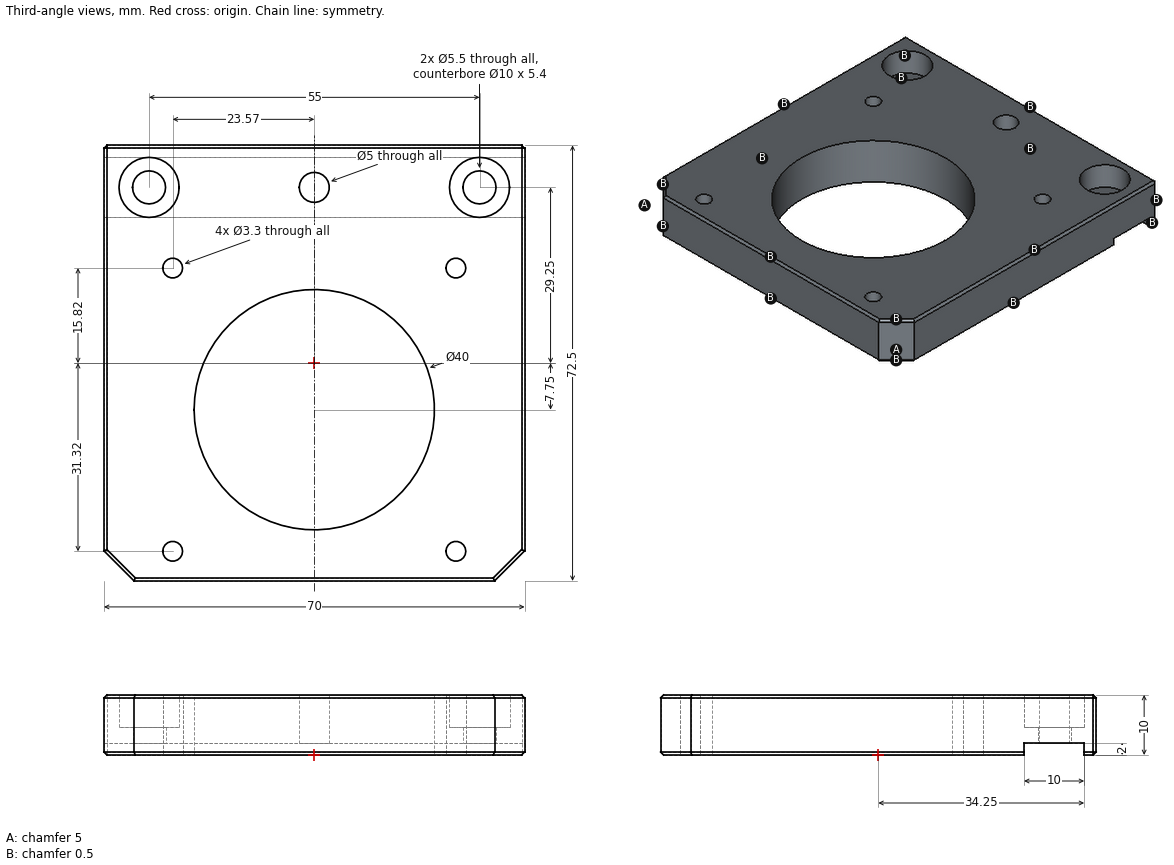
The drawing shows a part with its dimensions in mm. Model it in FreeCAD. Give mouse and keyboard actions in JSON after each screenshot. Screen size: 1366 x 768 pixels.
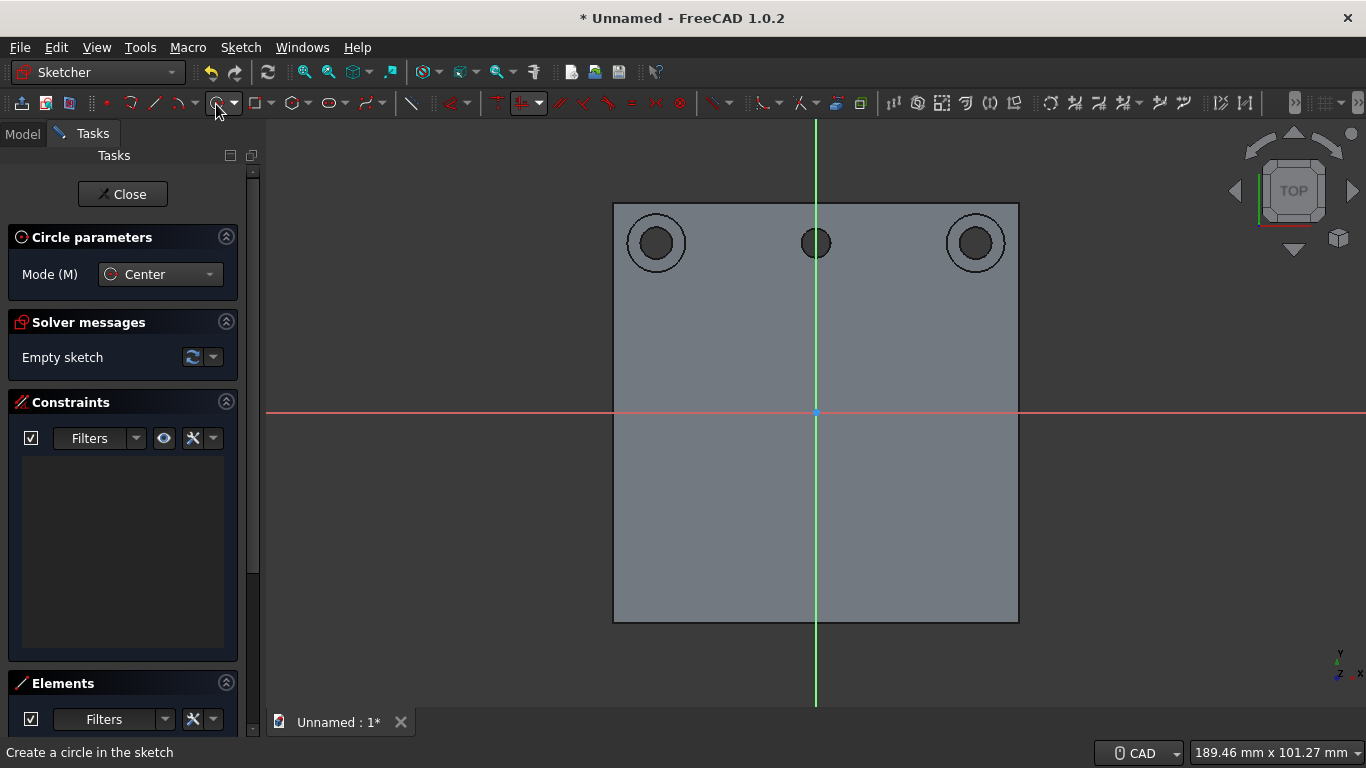
{"action": "scroll", "coordinate": [679, 321], "scroll_direction": "up", "scroll_amount": 5}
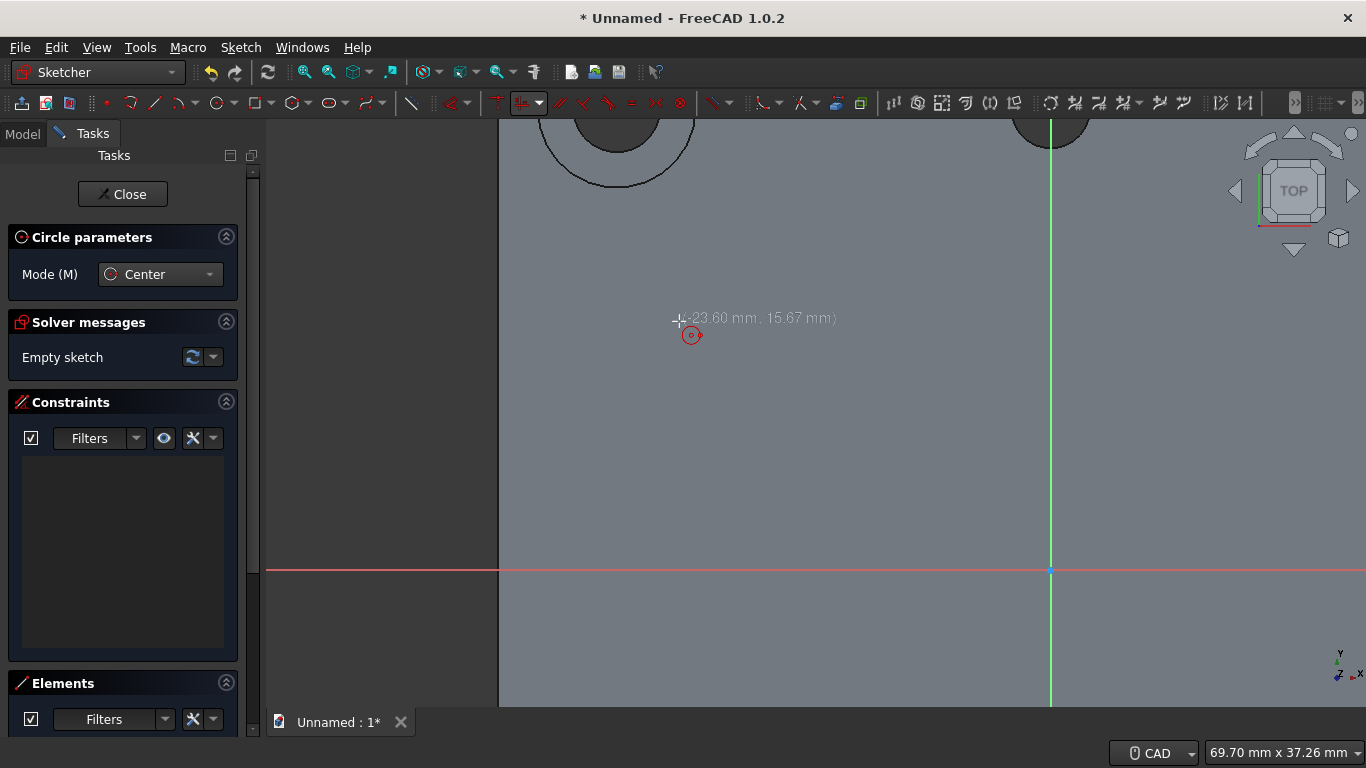
{"action": "left_click", "coordinate": [679, 321]}
{"action": "mouse_move", "coordinate": [697, 302]}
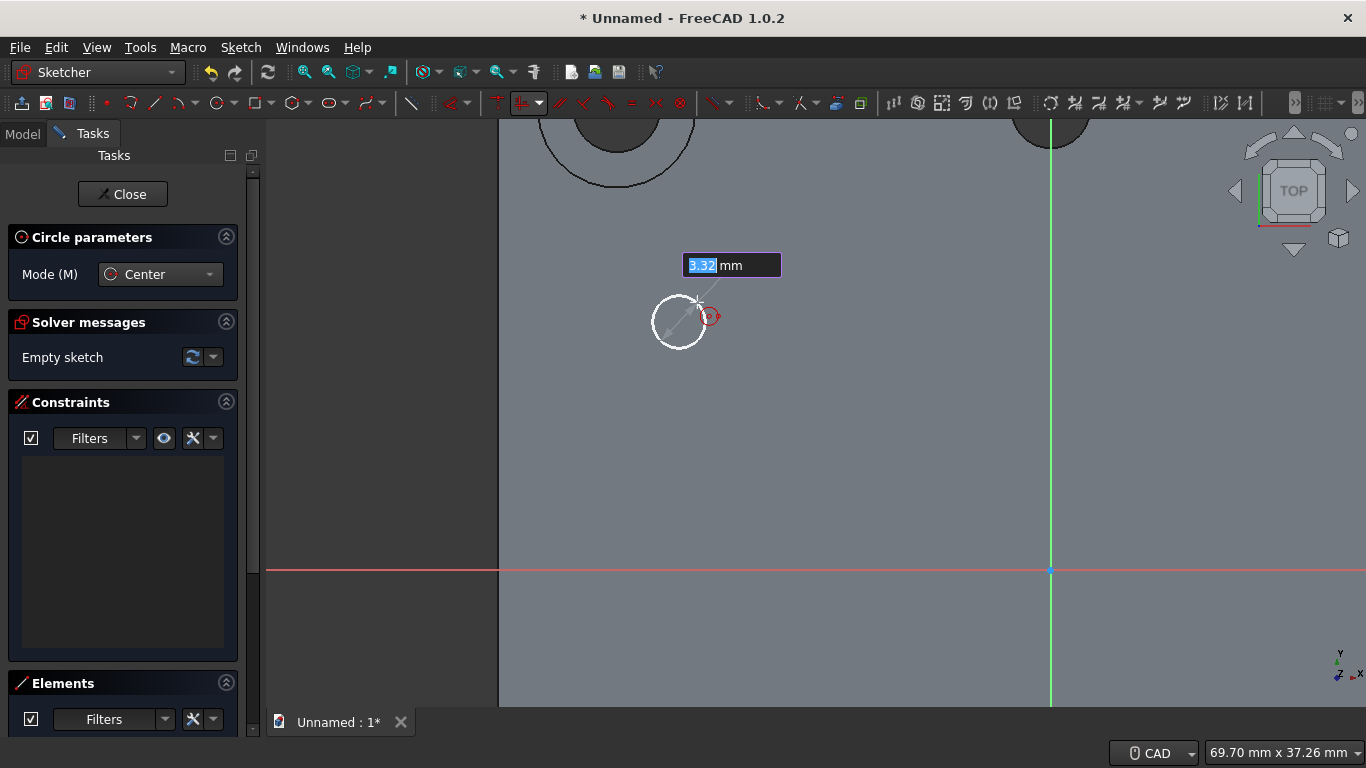
{"action": "type", "text": "3.3"}
{"action": "key", "text": "Return"}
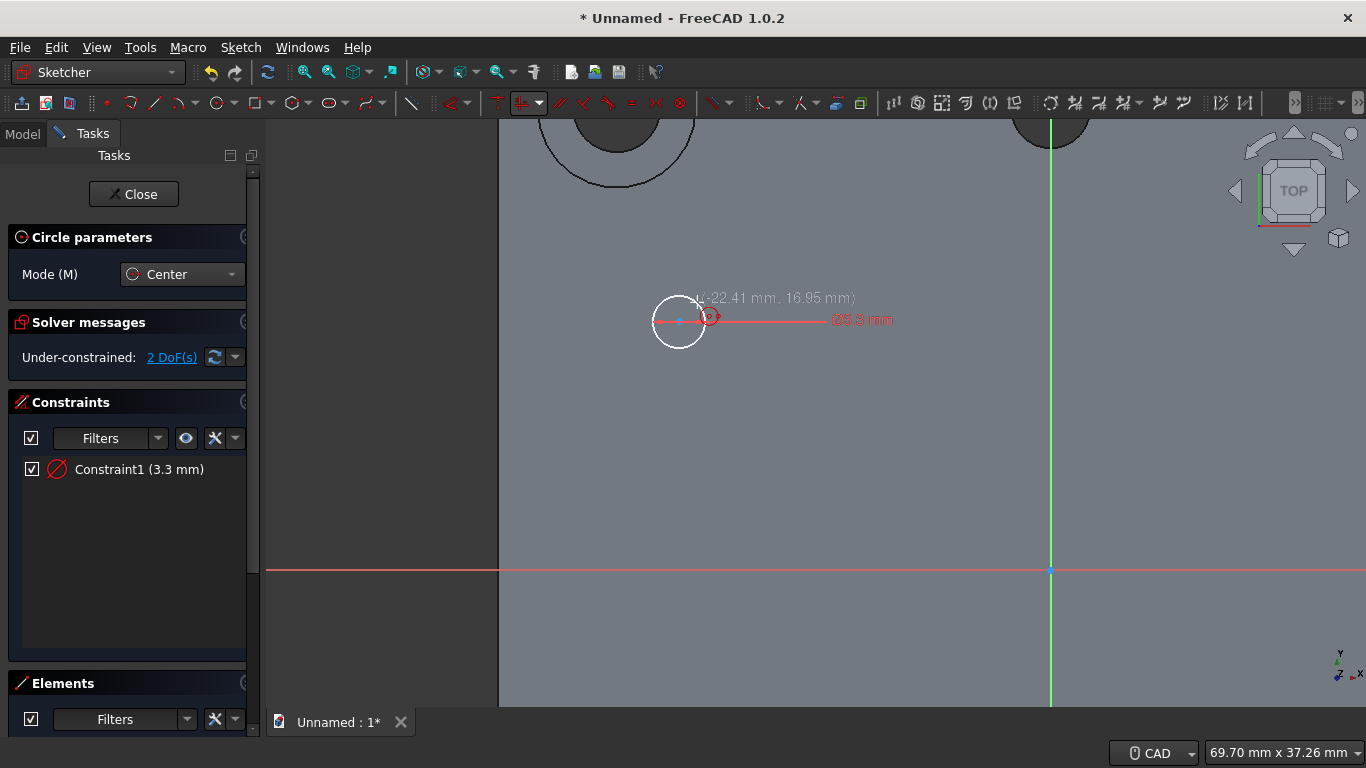
{"action": "scroll", "coordinate": [500, 185], "scroll_direction": "down", "scroll_amount": 4}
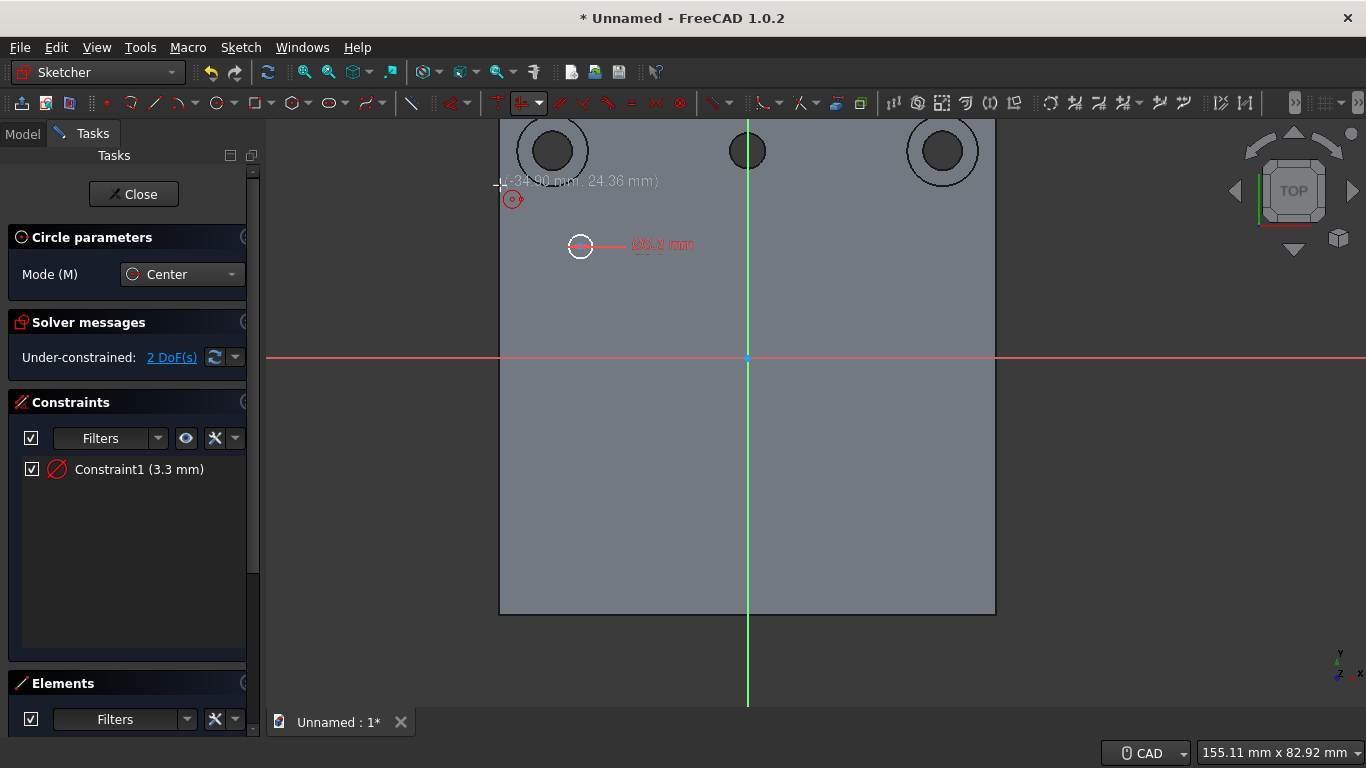
{"action": "scroll", "coordinate": [580, 580], "scroll_direction": "up", "scroll_amount": 4}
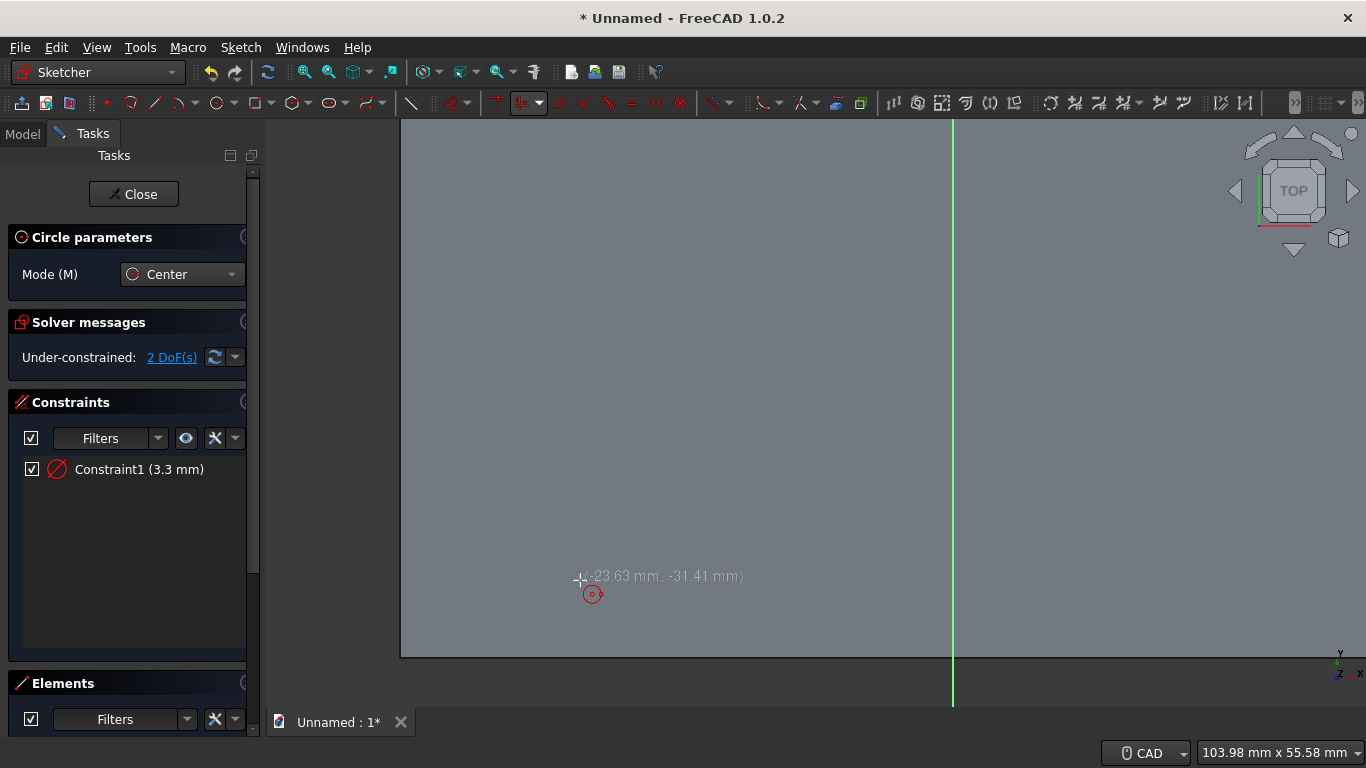
{"action": "left_click", "coordinate": [581, 580]}
{"action": "mouse_move", "coordinate": [599, 561]}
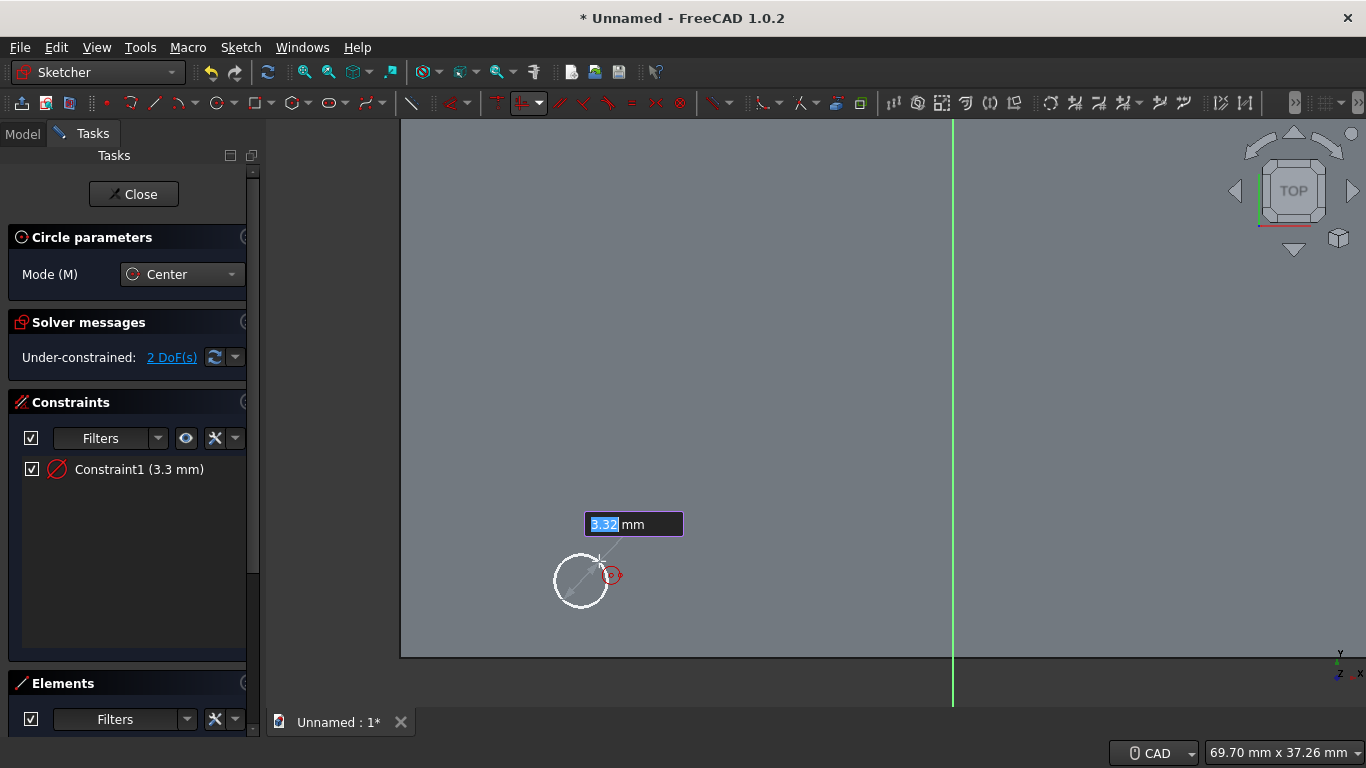
{"action": "type", "text": "3.3"}
{"action": "key", "text": "Return"}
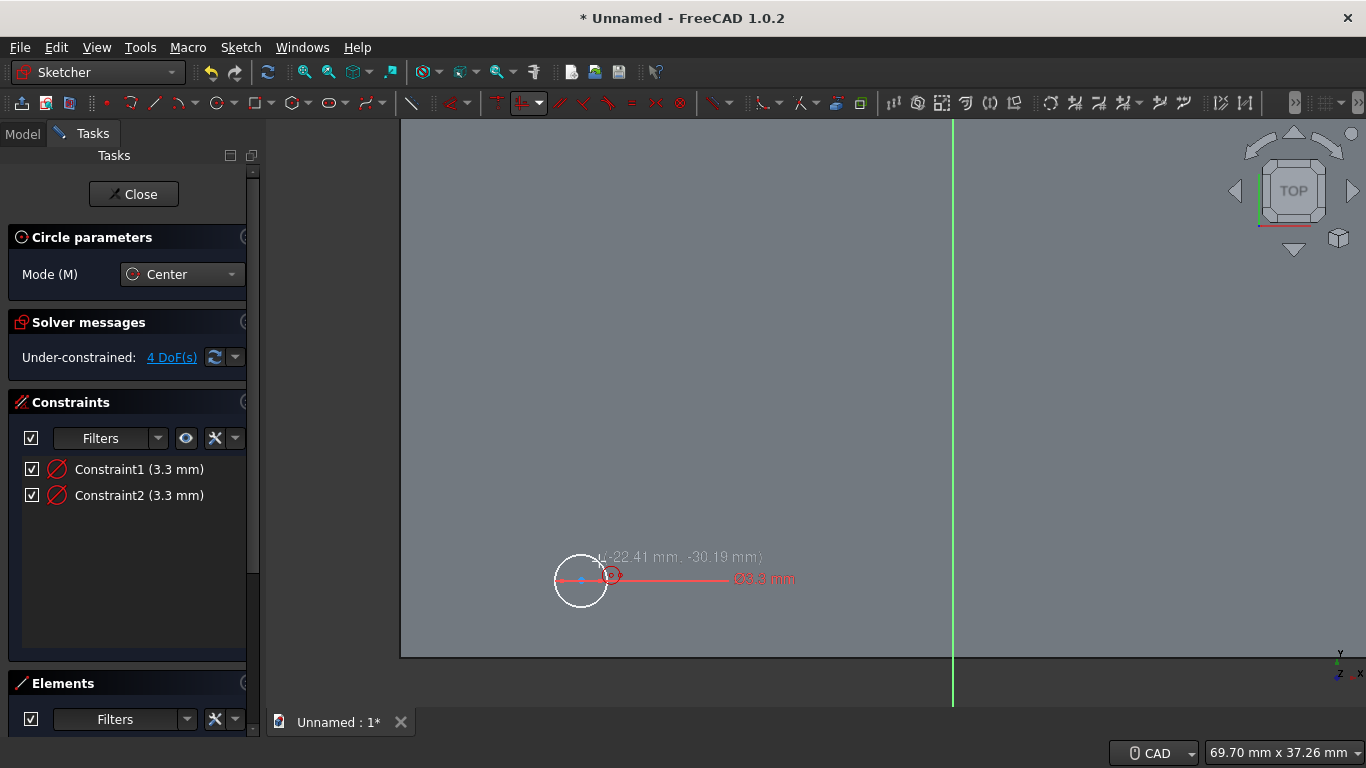
{"action": "scroll", "coordinate": [580, 580], "scroll_direction": "down", "scroll_amount": 4}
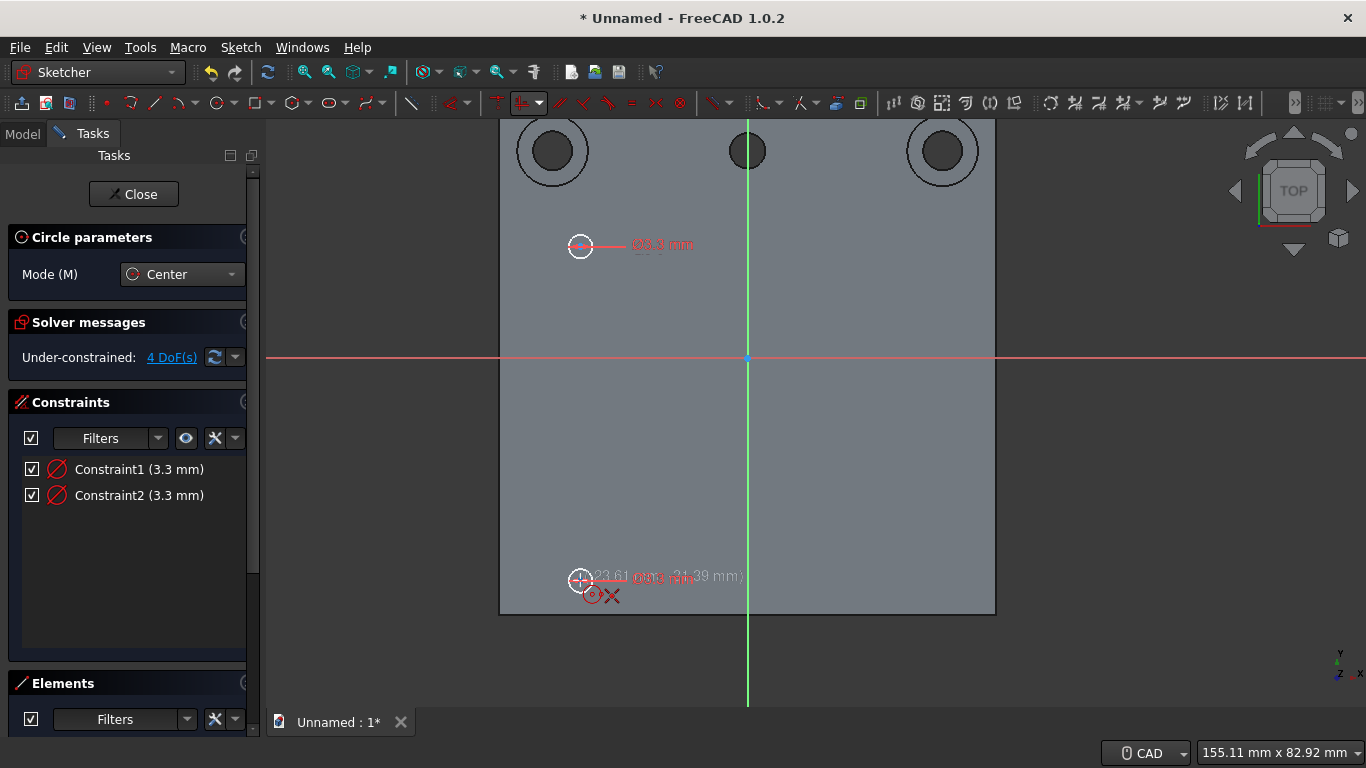
{"action": "scroll", "coordinate": [915, 580], "scroll_direction": "up", "scroll_amount": 4}